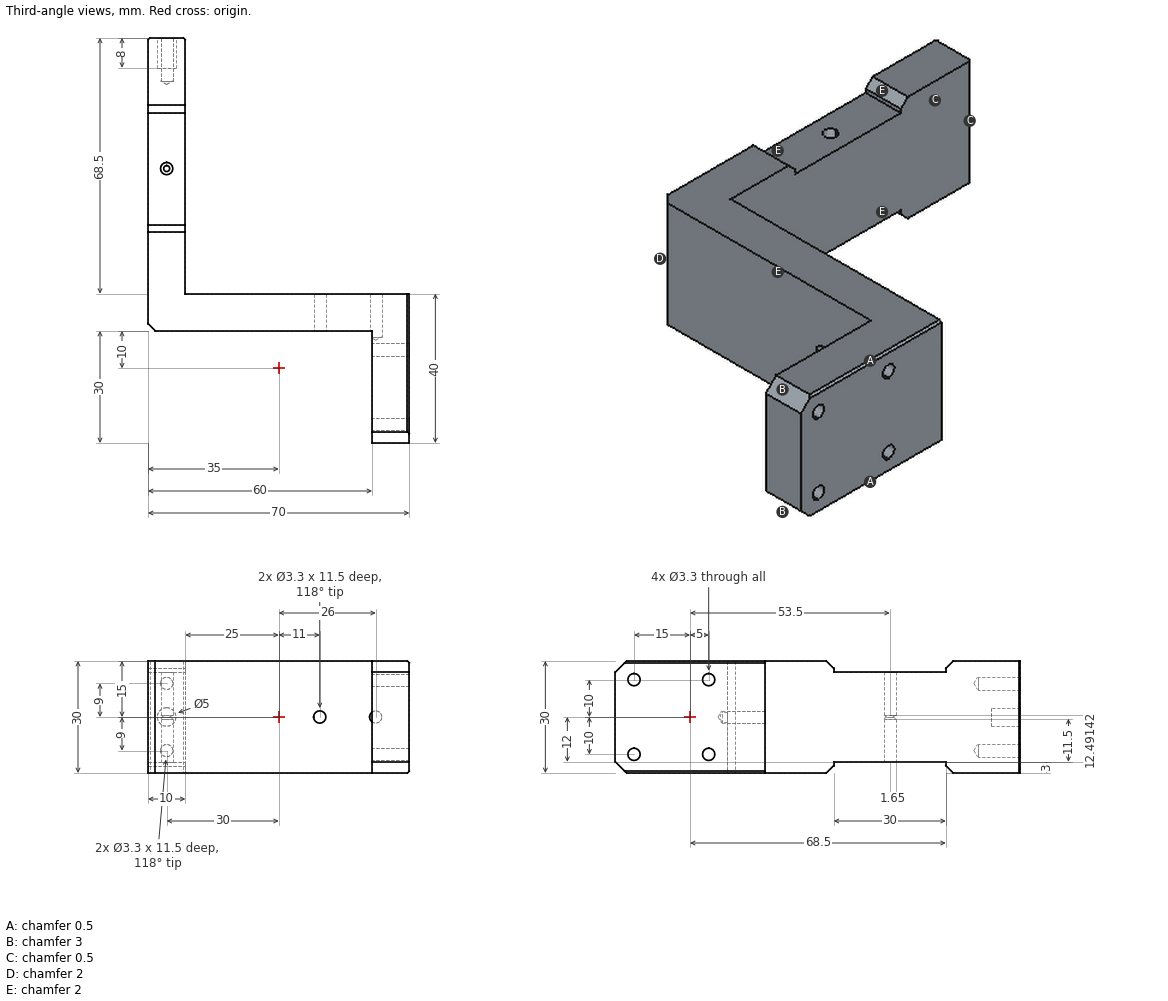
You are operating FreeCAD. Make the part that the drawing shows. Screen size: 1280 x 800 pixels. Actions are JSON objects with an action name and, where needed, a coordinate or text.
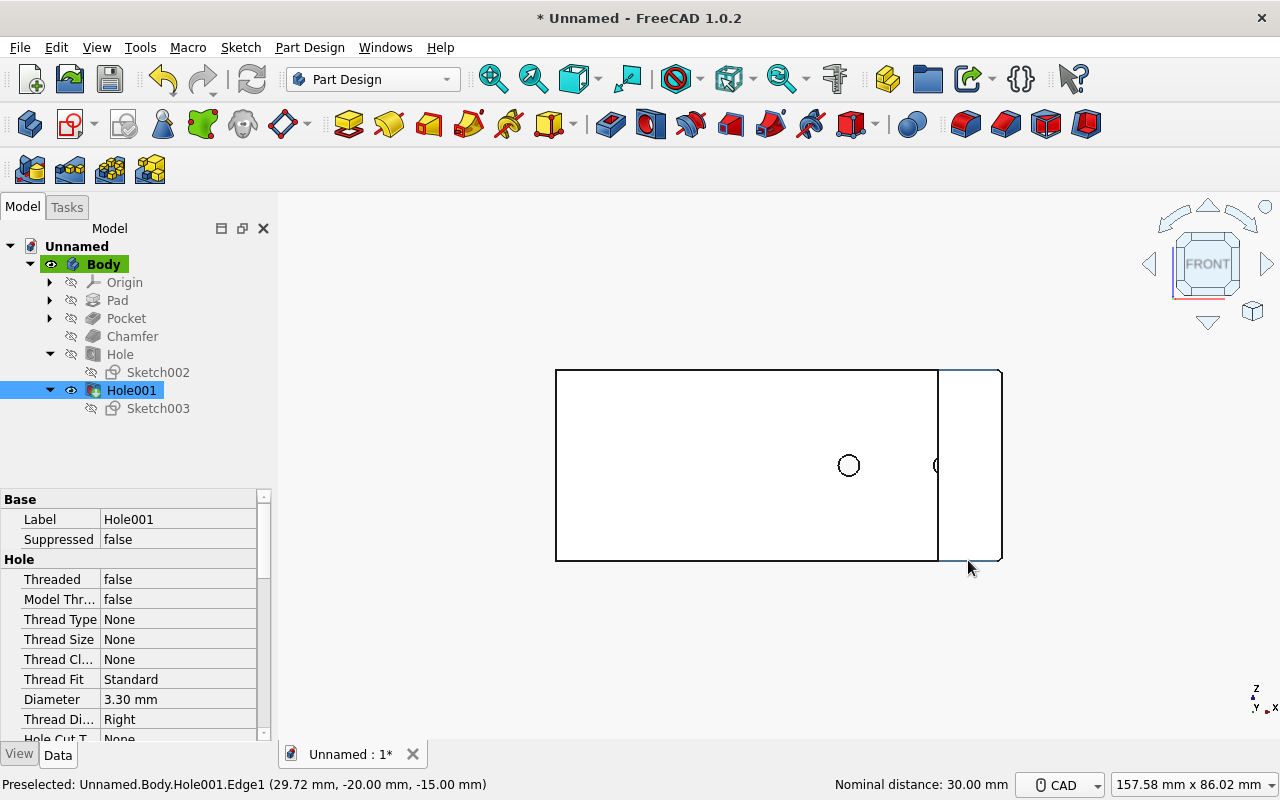
{"action": "left_click", "coordinate": [1006, 124]}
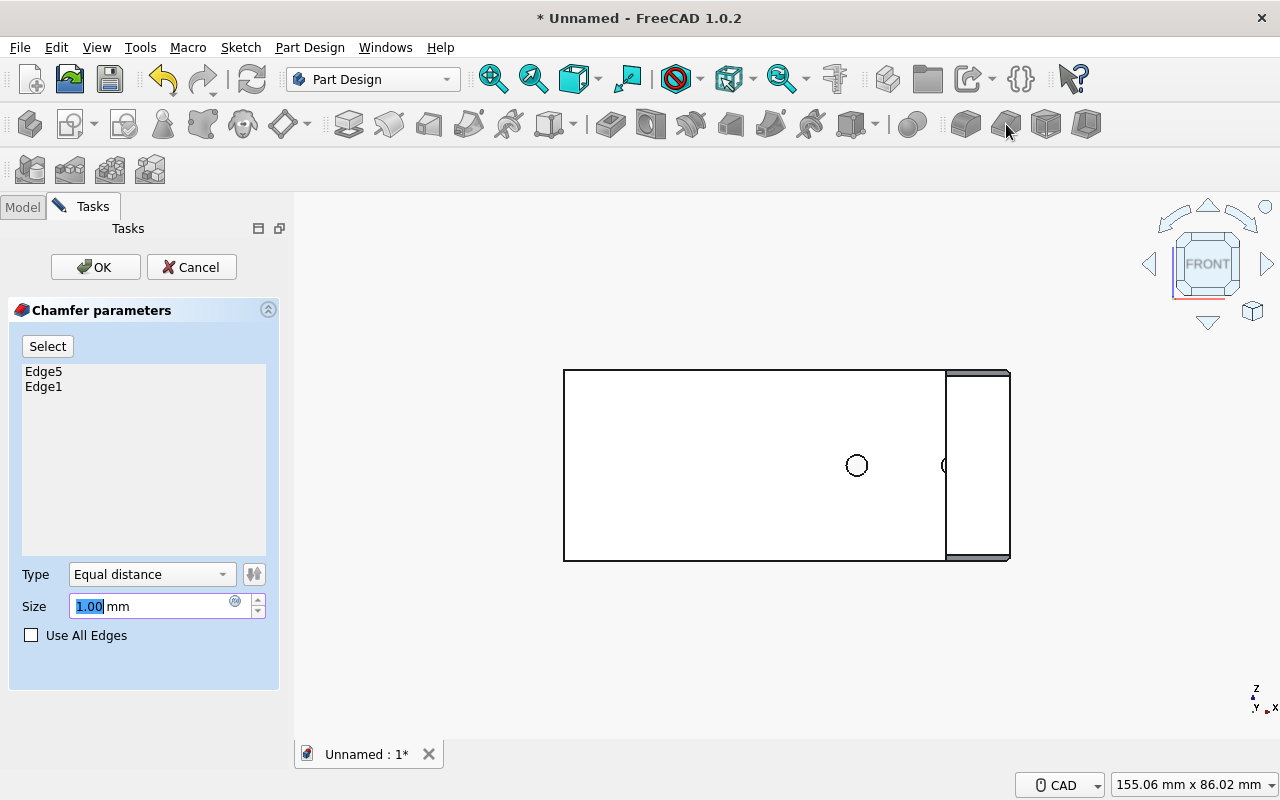
{"action": "type", "text": "3"}
{"action": "key", "text": "Tab"}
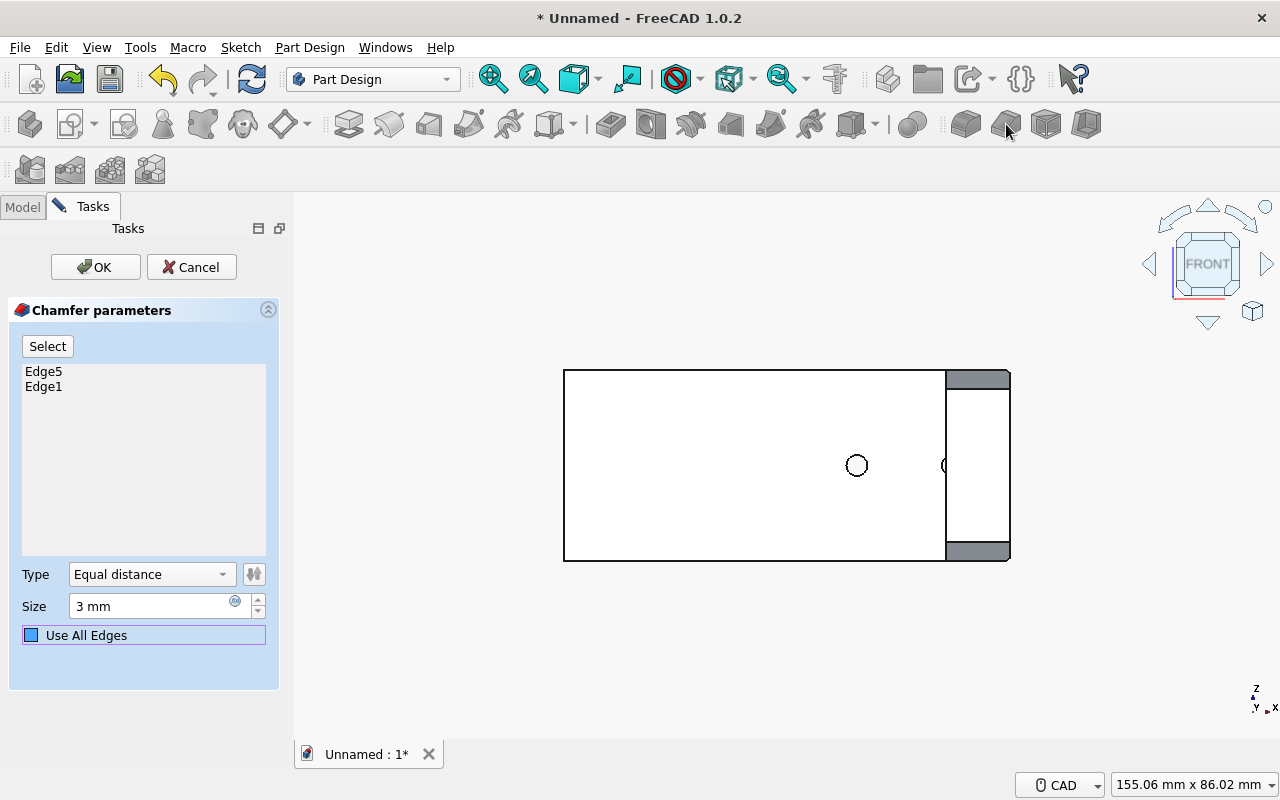
{"action": "left_click", "coordinate": [96, 267]}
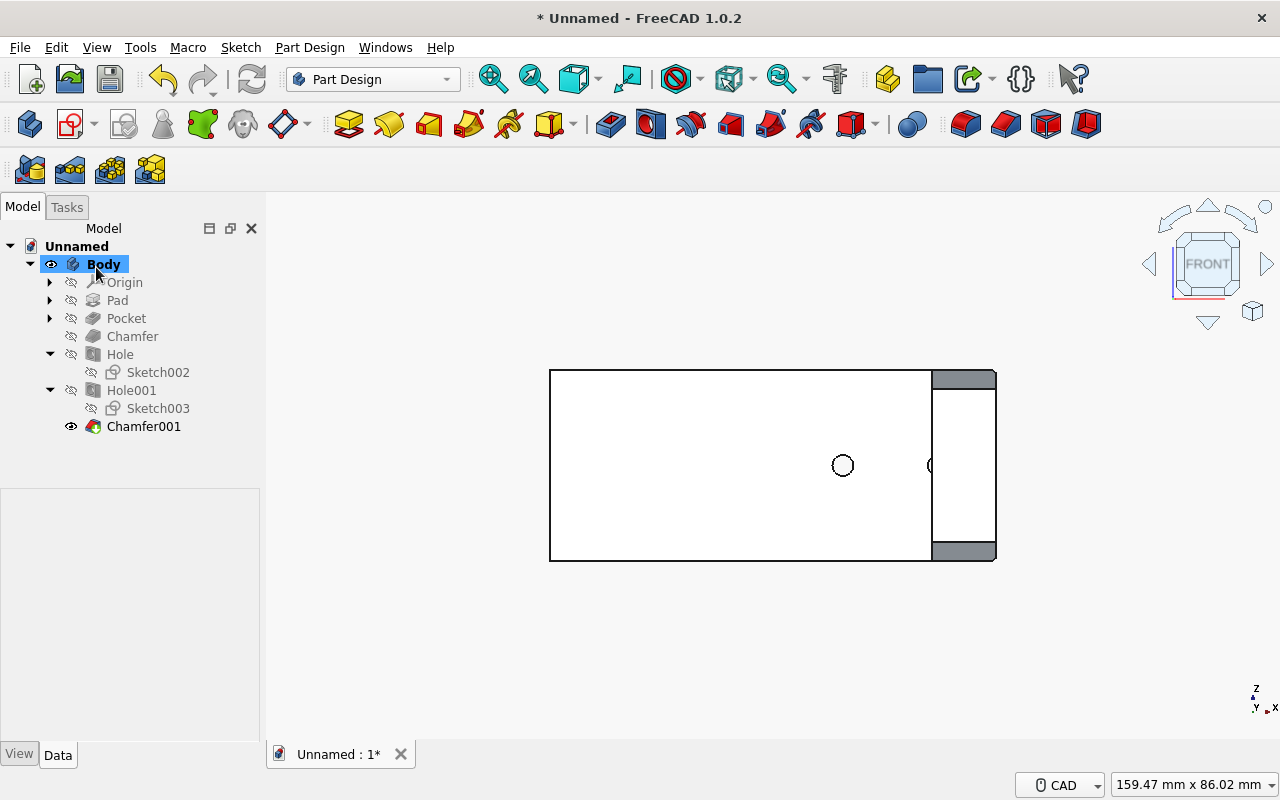
{"action": "left_click", "coordinate": [494, 80]}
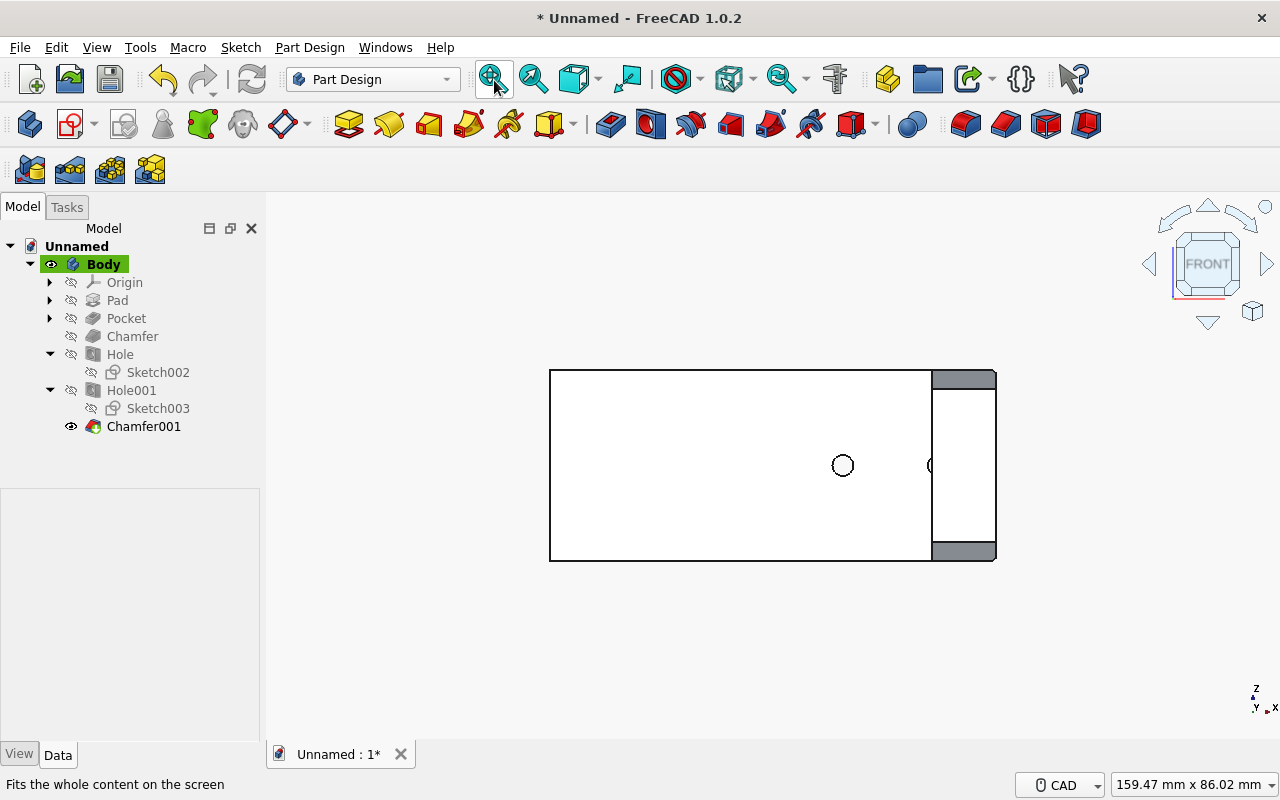
{"action": "key", "text": "4"}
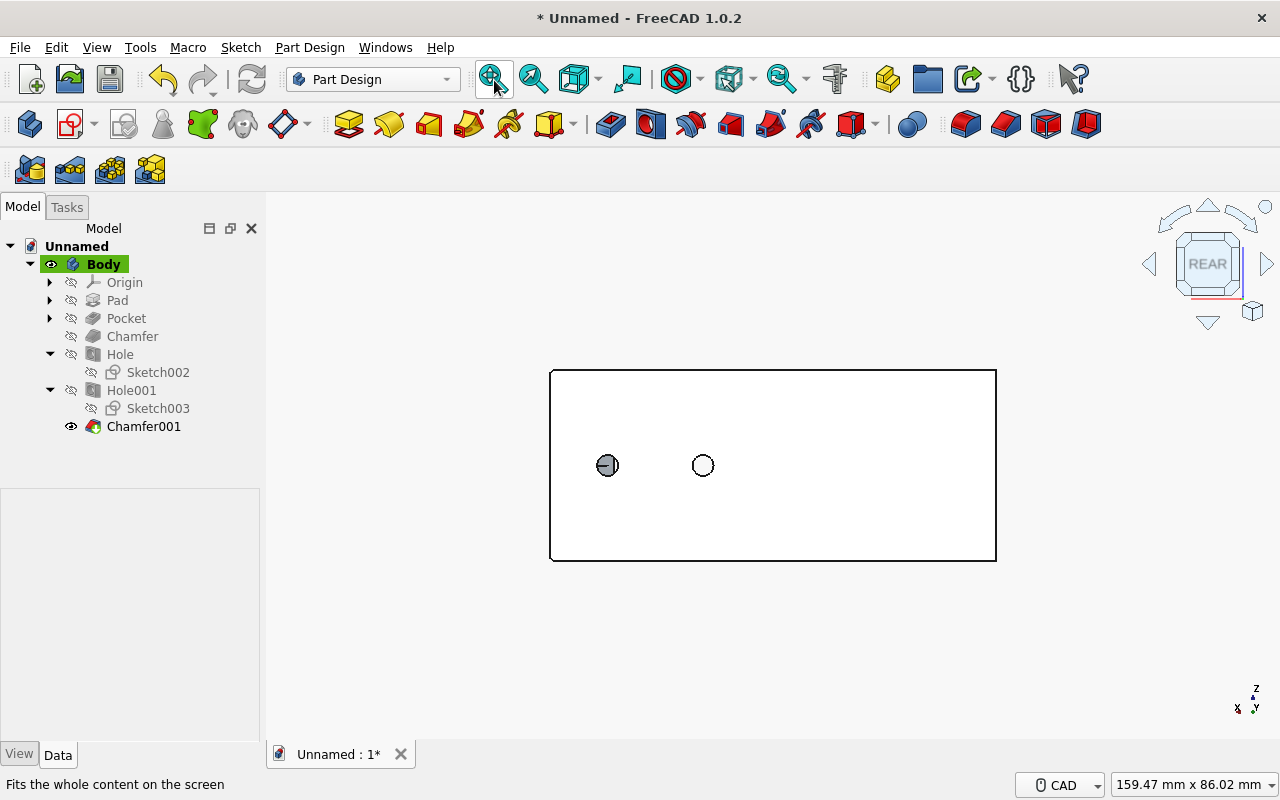
{"action": "key", "text": "v f"}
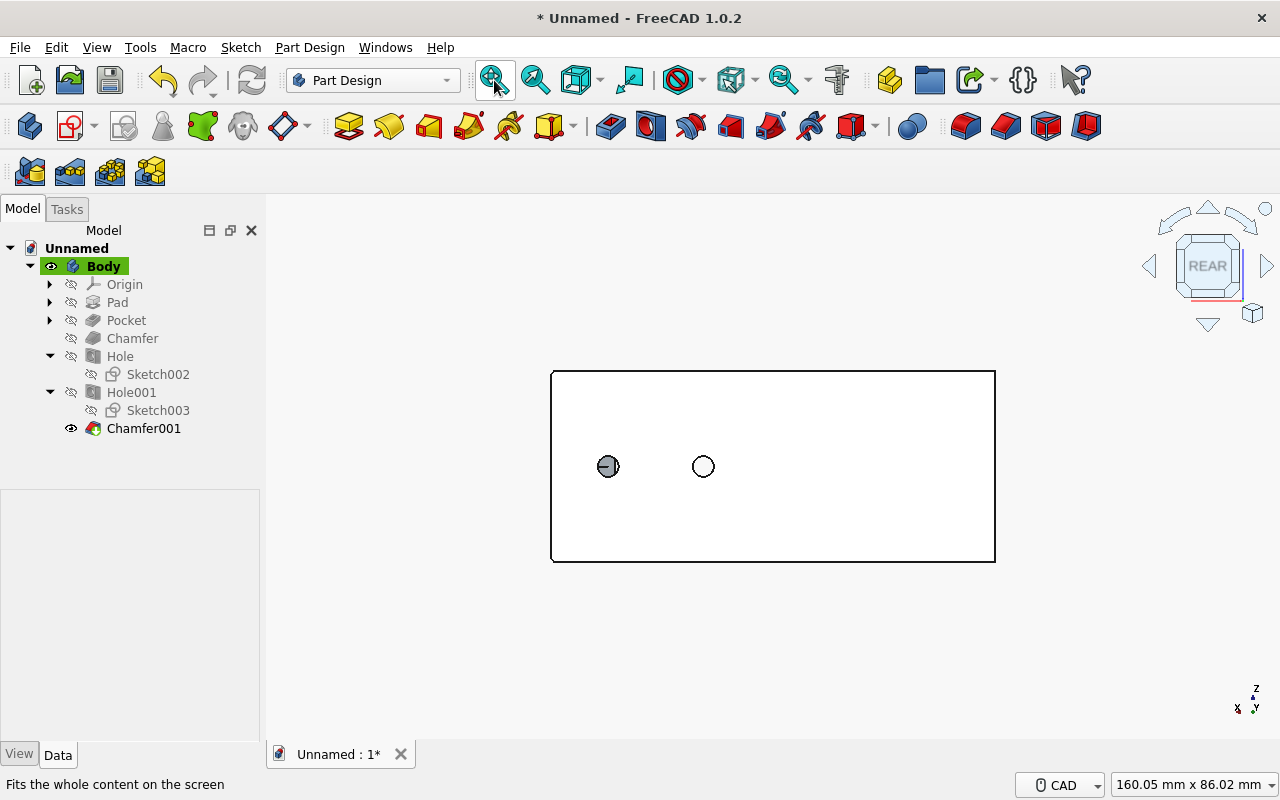
{"action": "left_click", "coordinate": [836, 466]}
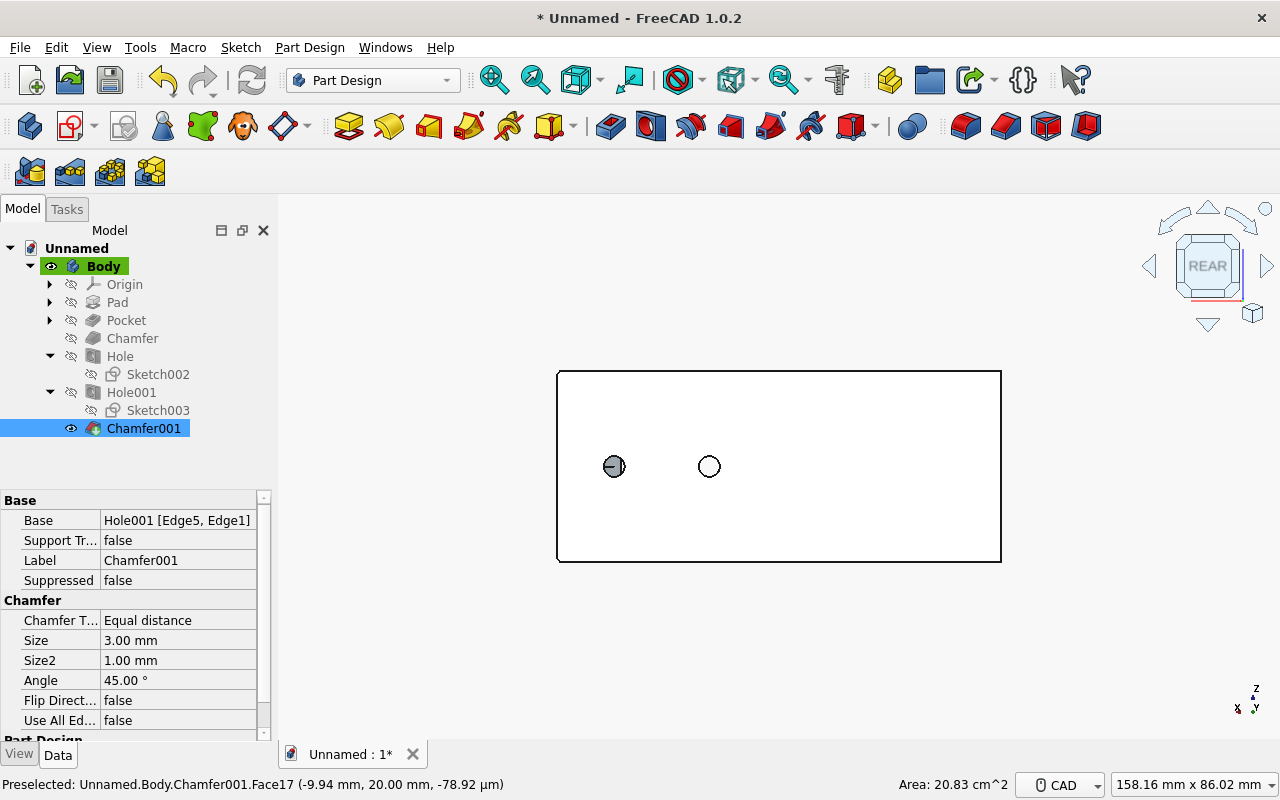
{"action": "left_click", "coordinate": [70, 126]}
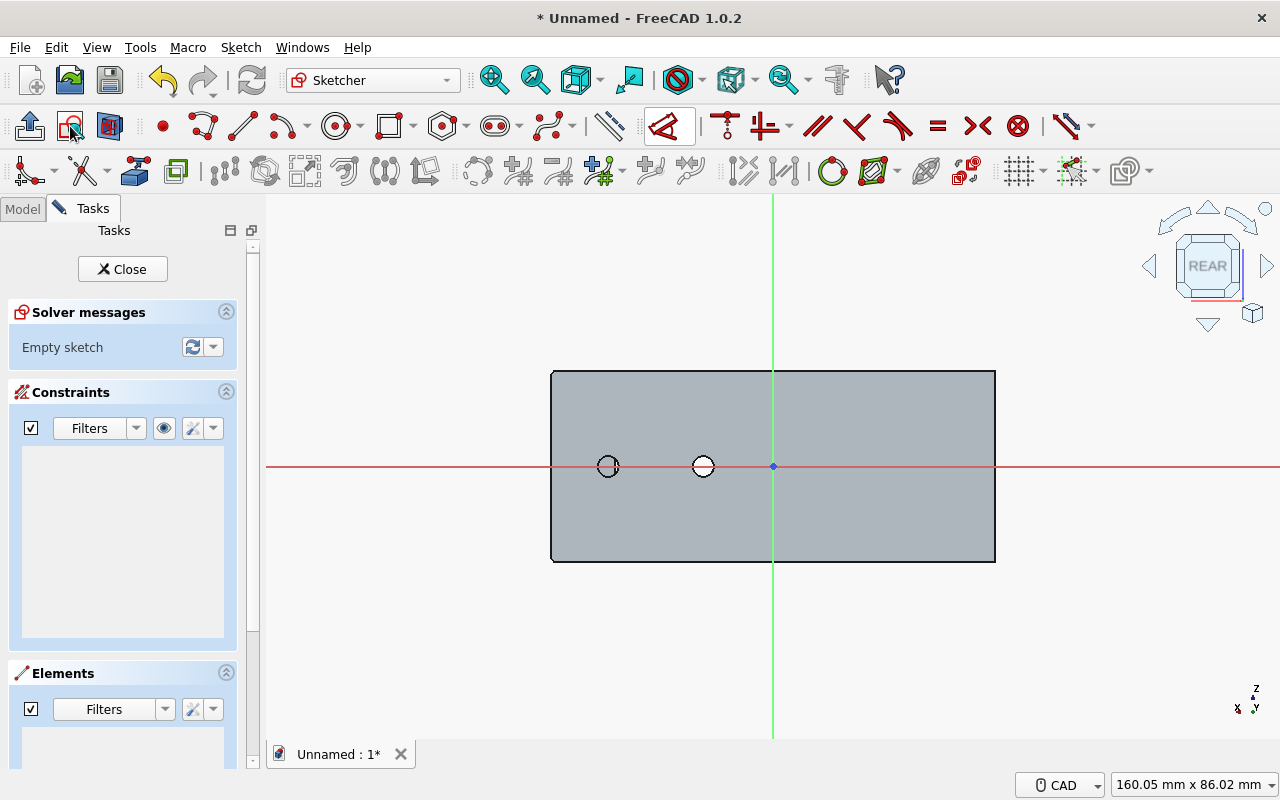
{"action": "scroll", "coordinate": [1102, 466], "scroll_direction": "up", "scroll_amount": 3}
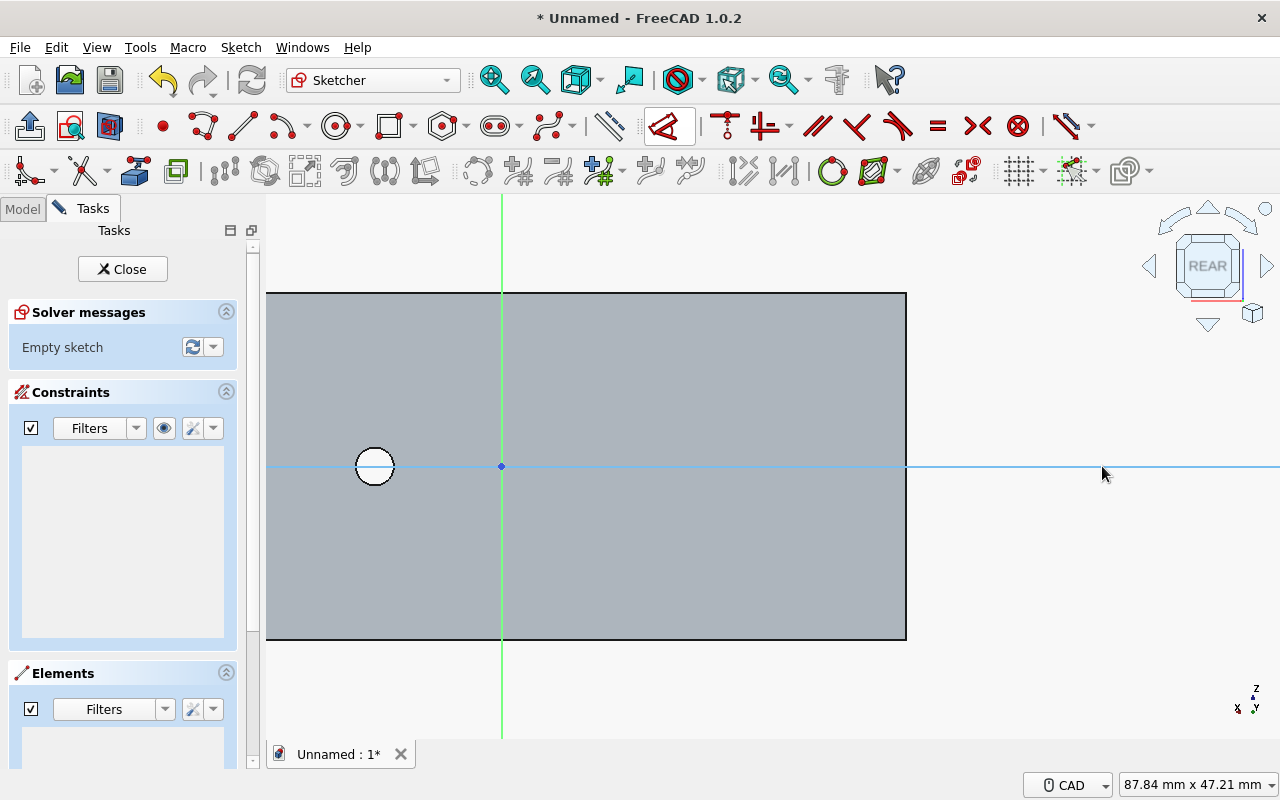
{"action": "left_click", "coordinate": [390, 126]}